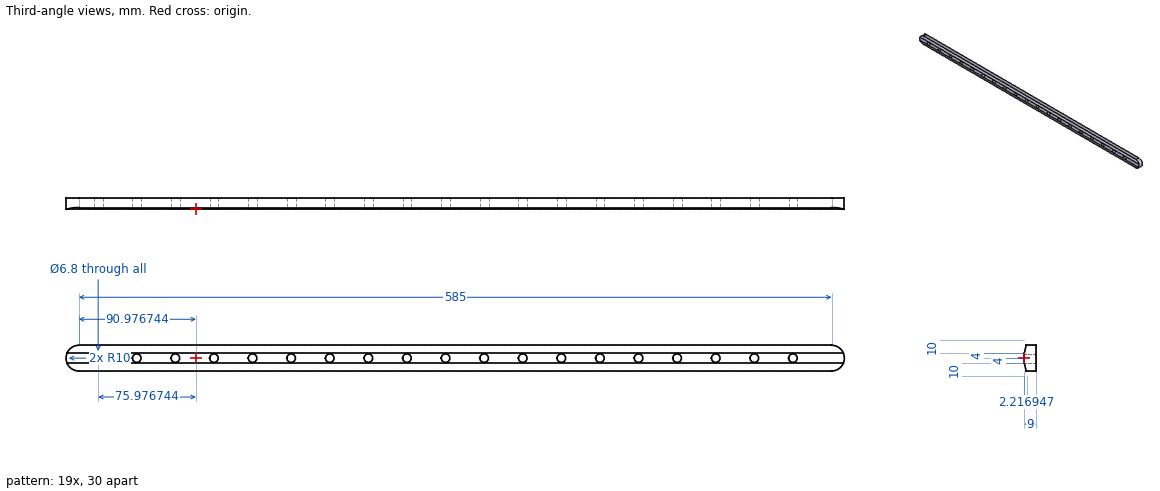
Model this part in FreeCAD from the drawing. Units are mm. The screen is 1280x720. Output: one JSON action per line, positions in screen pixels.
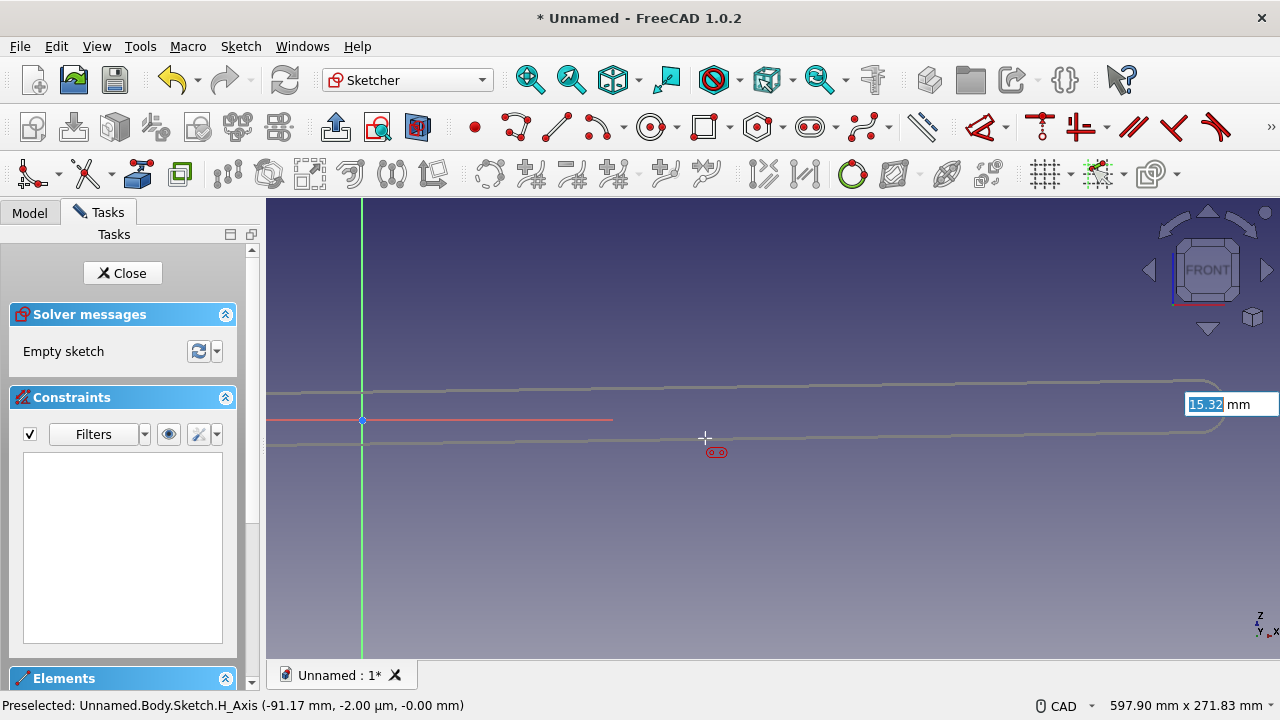
{"action": "left_click", "coordinate": [704, 437]}
{"action": "key", "text": "Escape"}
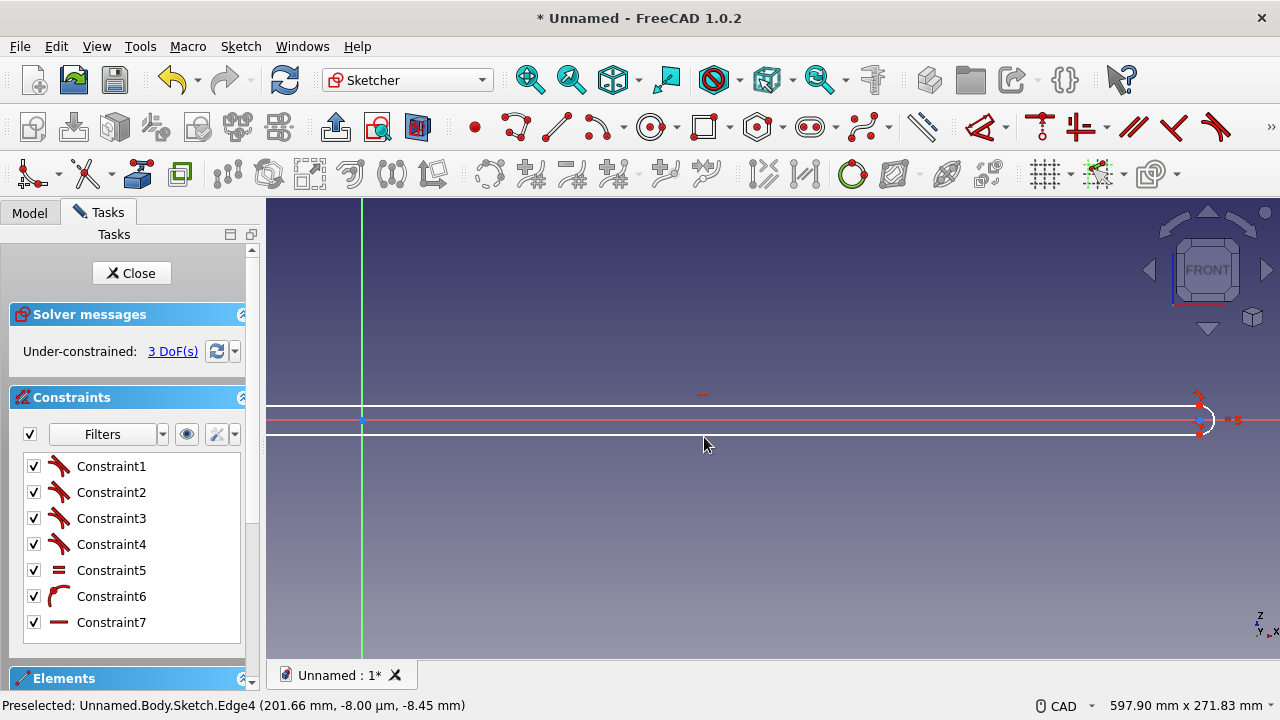
{"action": "left_click", "coordinate": [980, 128]}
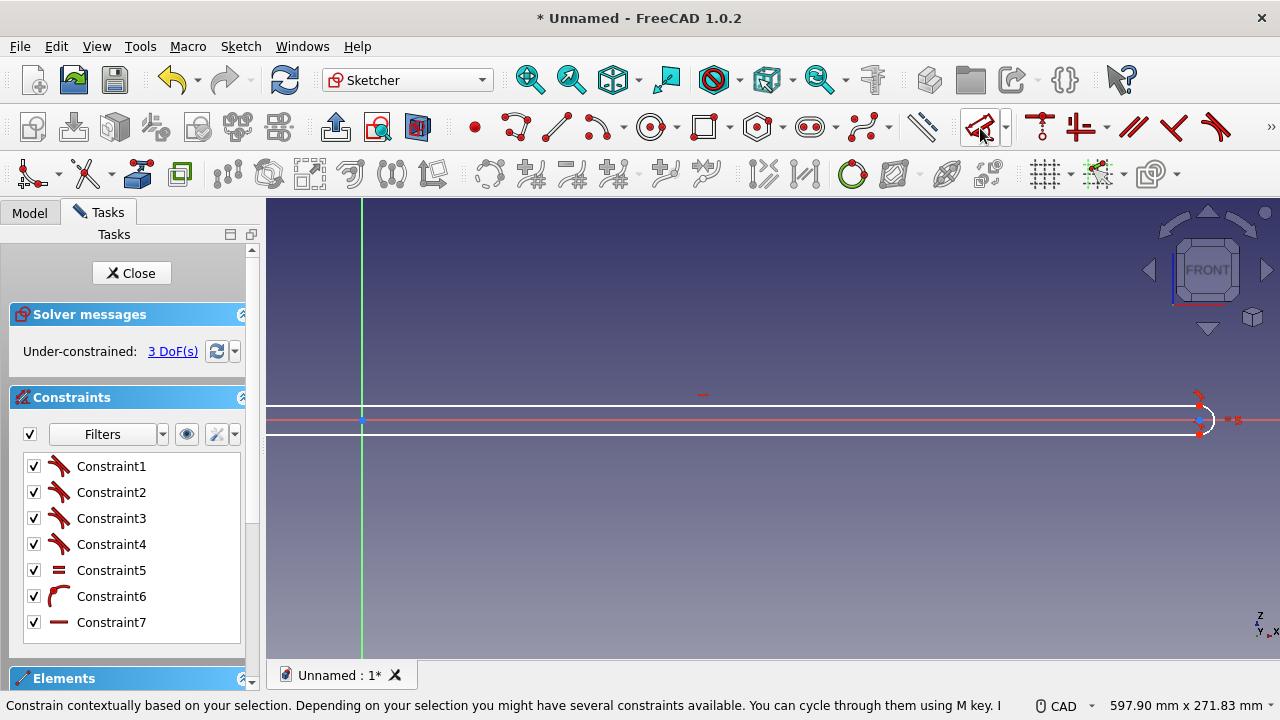
{"action": "scroll", "coordinate": [705, 439], "scroll_direction": "down", "scroll_amount": 3}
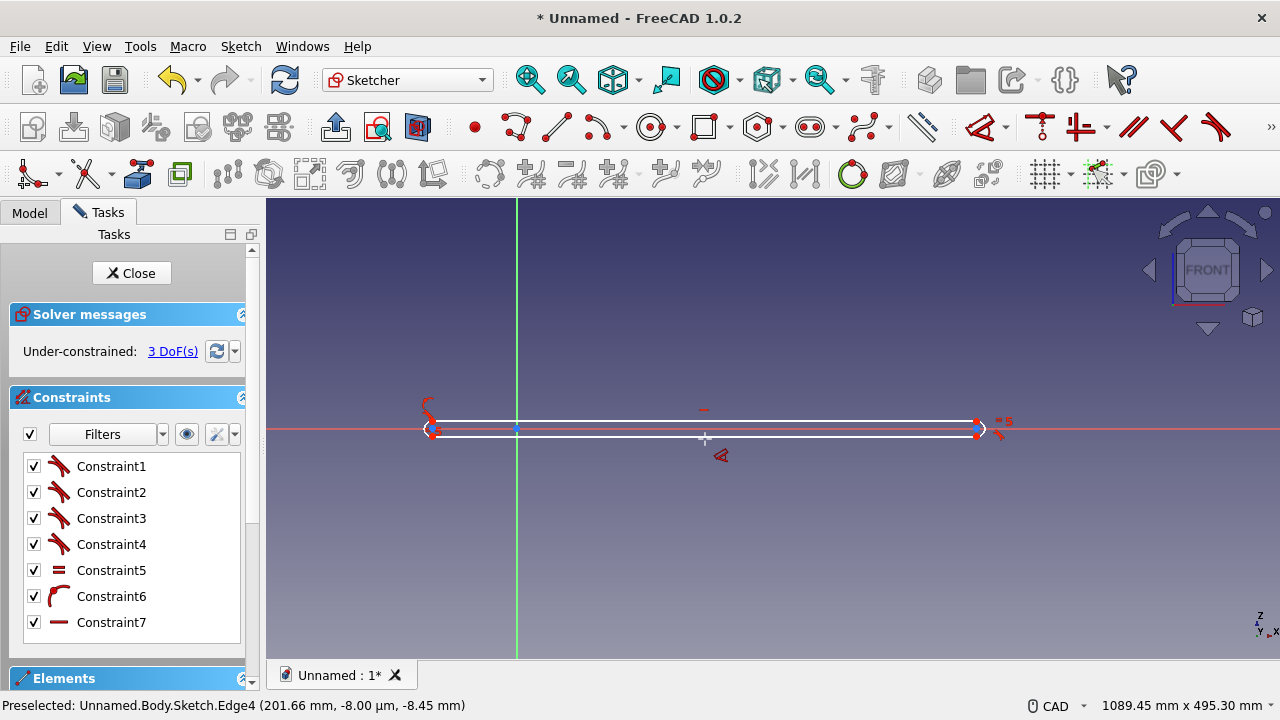
{"action": "scroll", "coordinate": [424, 429], "scroll_direction": "up", "scroll_amount": 8}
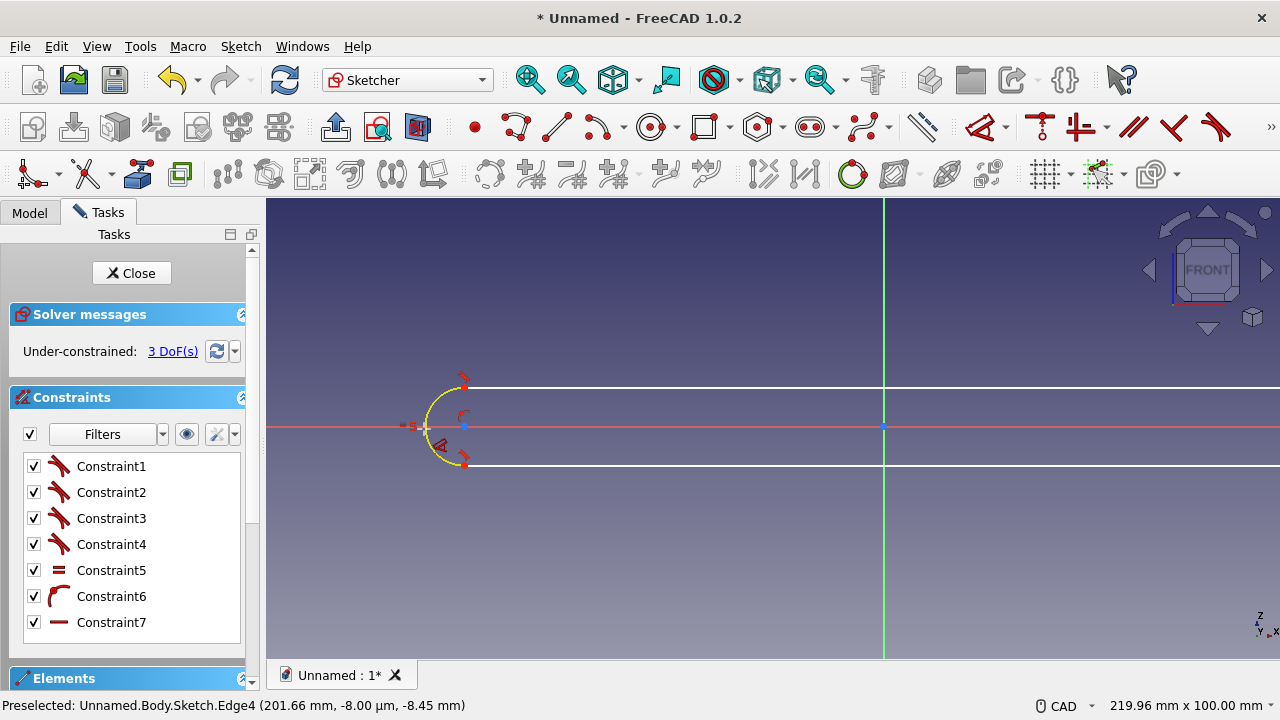
{"action": "left_click", "coordinate": [426, 427]}
{"action": "left_click", "coordinate": [402, 393]}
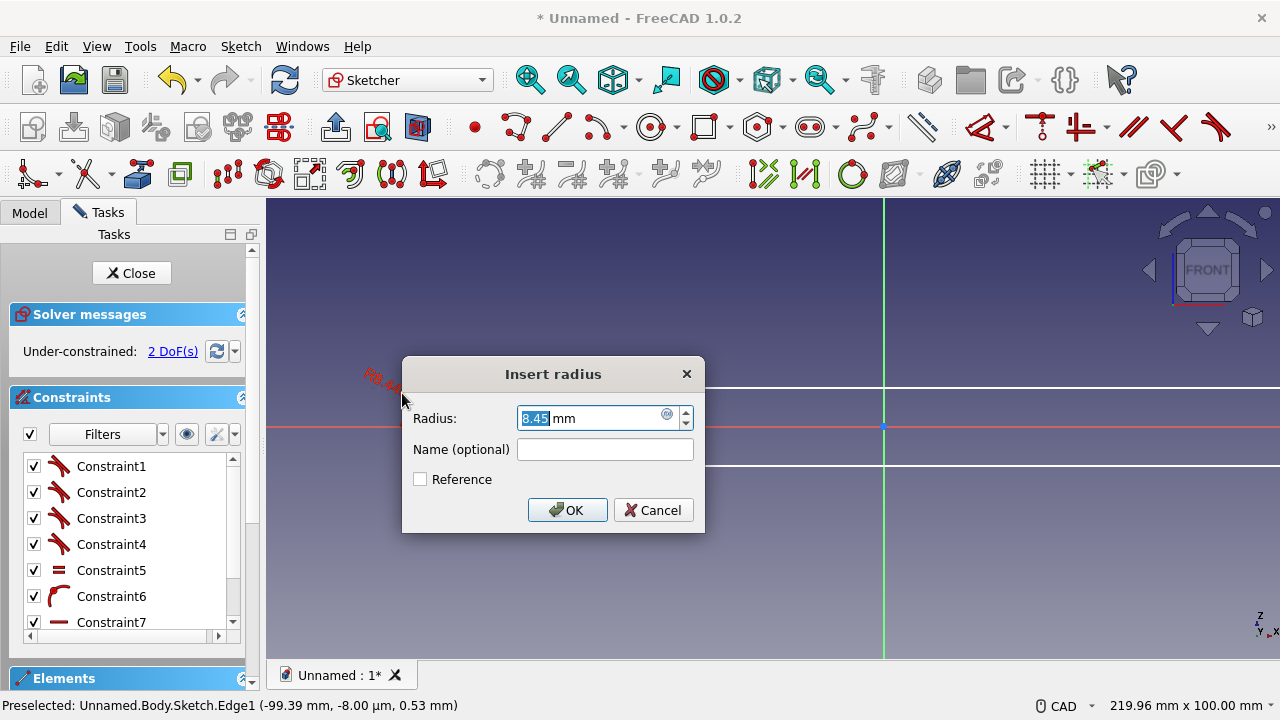
{"action": "type", "text": "10"}
{"action": "key", "text": "Return"}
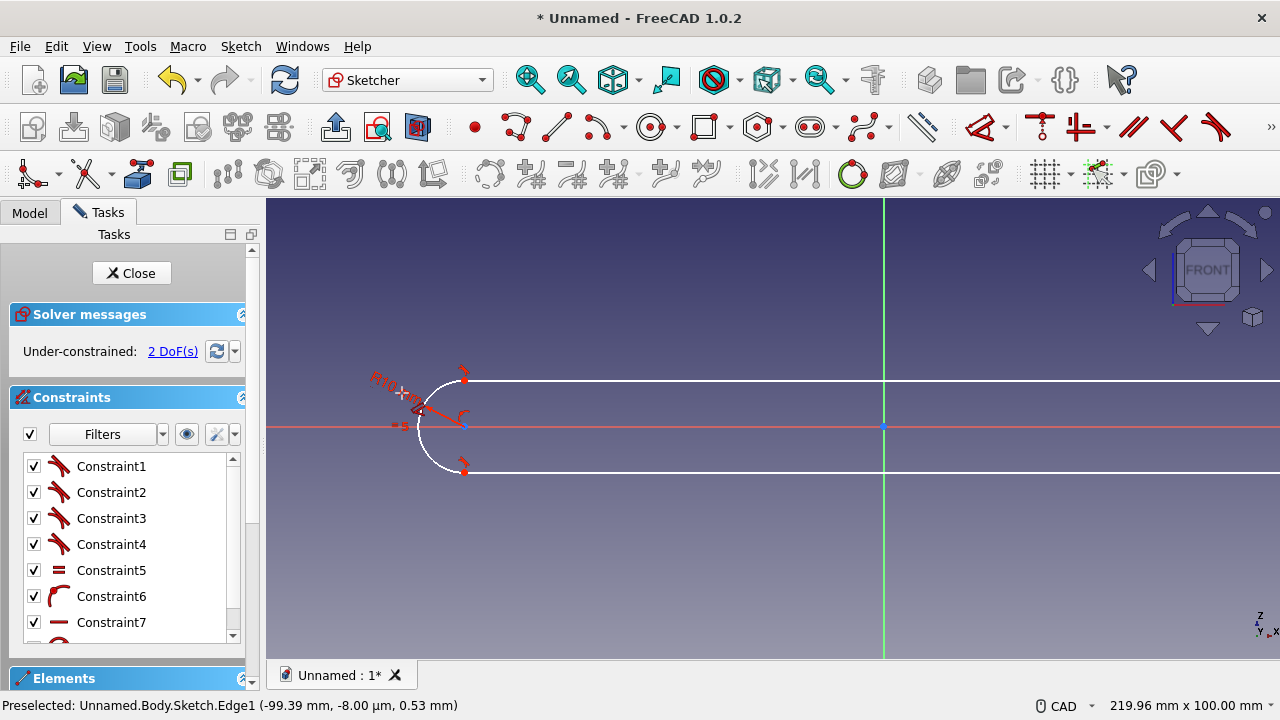
{"action": "scroll", "coordinate": [424, 429], "scroll_direction": "down", "scroll_amount": 8}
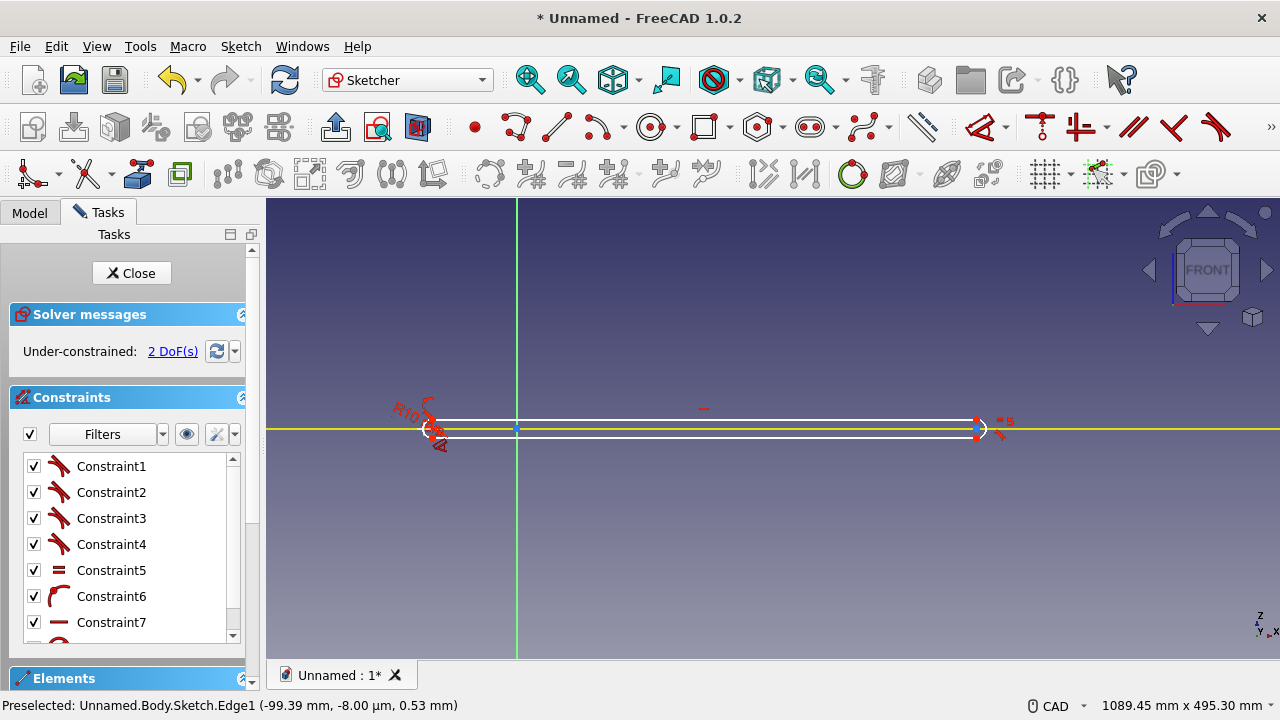
{"action": "scroll", "coordinate": [541, 420], "scroll_direction": "up", "scroll_amount": 2}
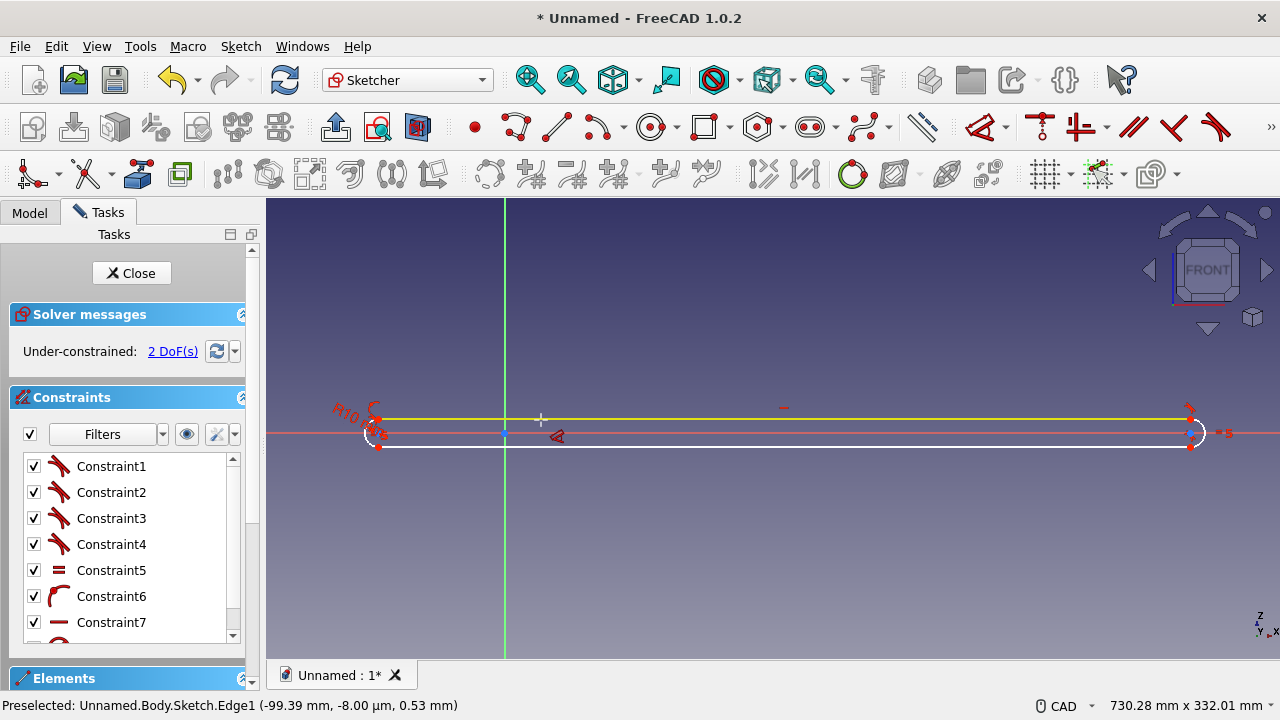
{"action": "left_click", "coordinate": [541, 419]}
{"action": "left_click", "coordinate": [747, 385]}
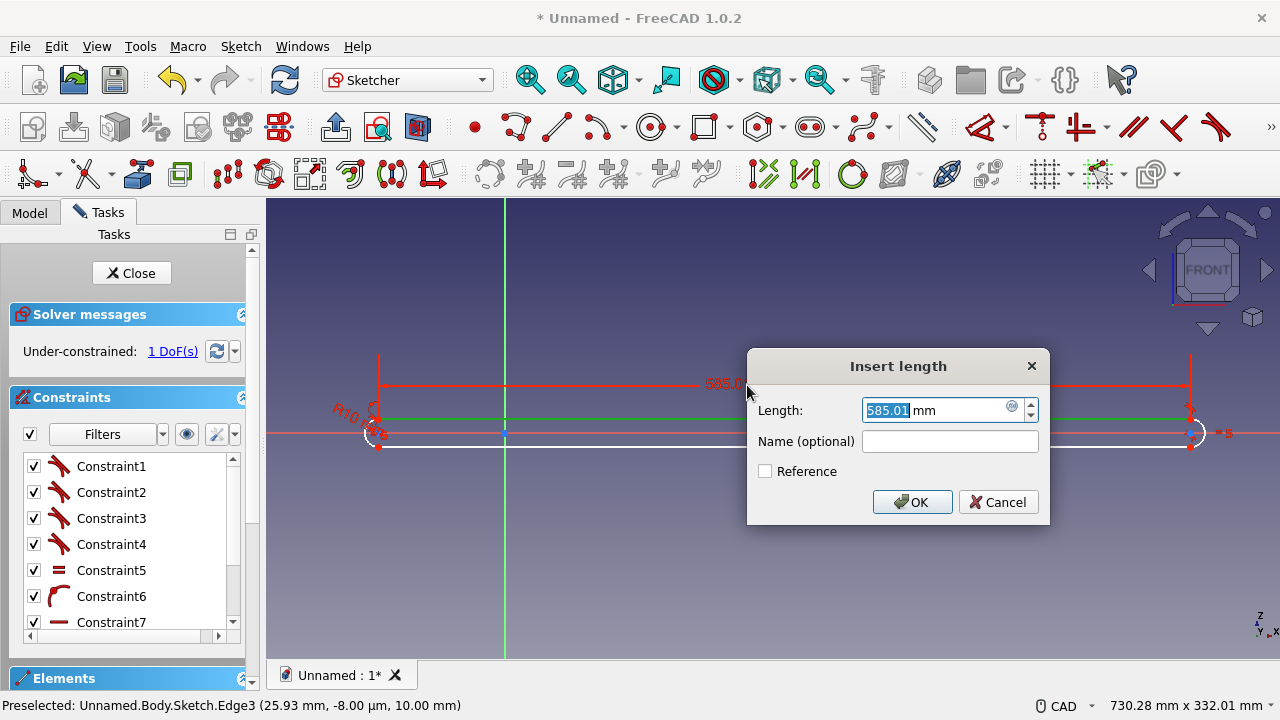
{"action": "type", "text": "585"}
{"action": "key", "text": "Return"}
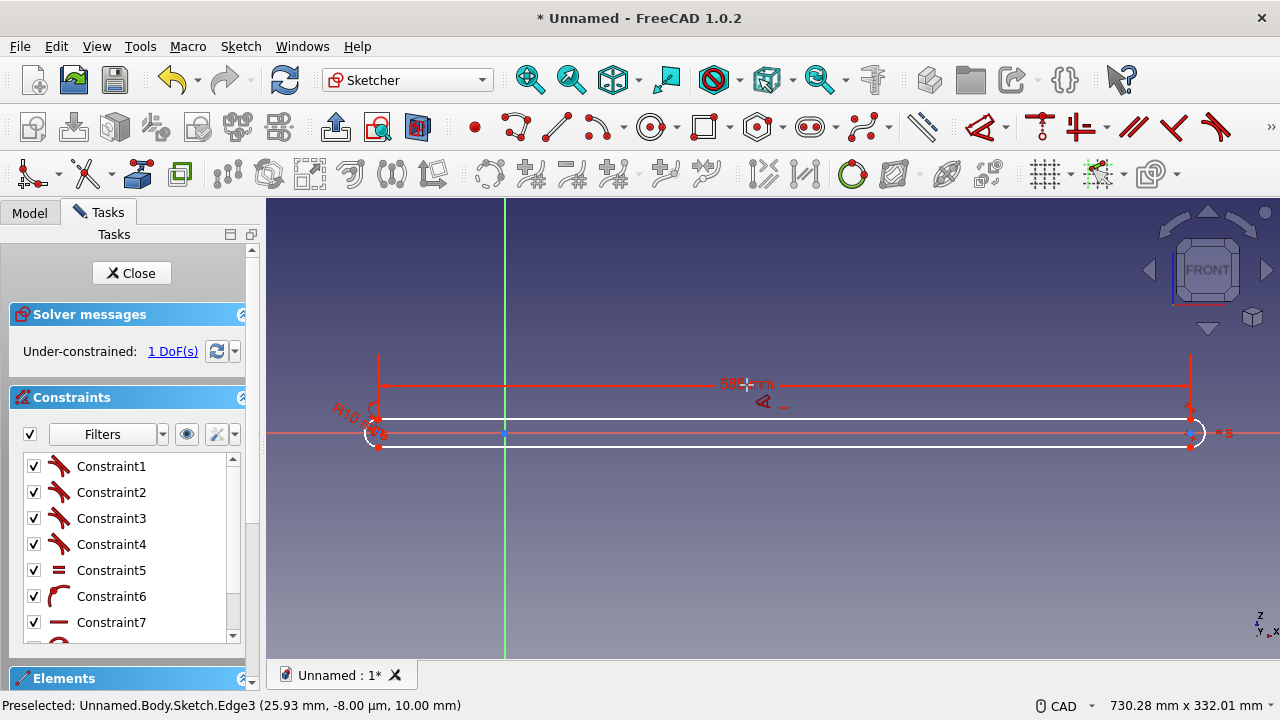
{"action": "left_click", "coordinate": [379, 419]}
{"action": "left_click", "coordinate": [442, 385]}